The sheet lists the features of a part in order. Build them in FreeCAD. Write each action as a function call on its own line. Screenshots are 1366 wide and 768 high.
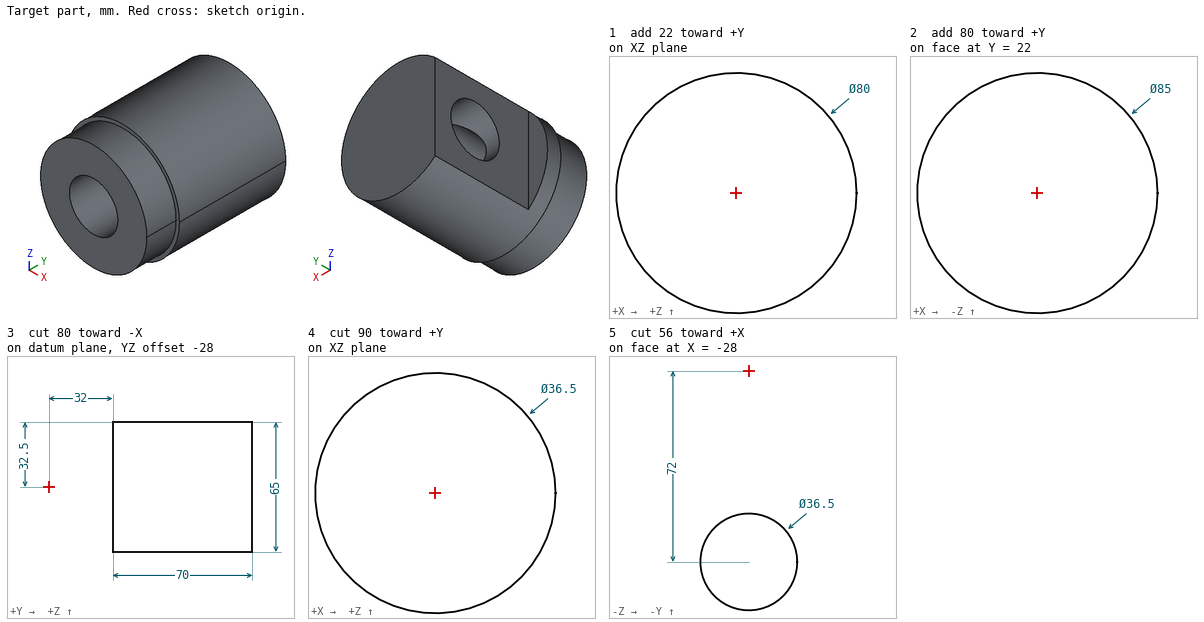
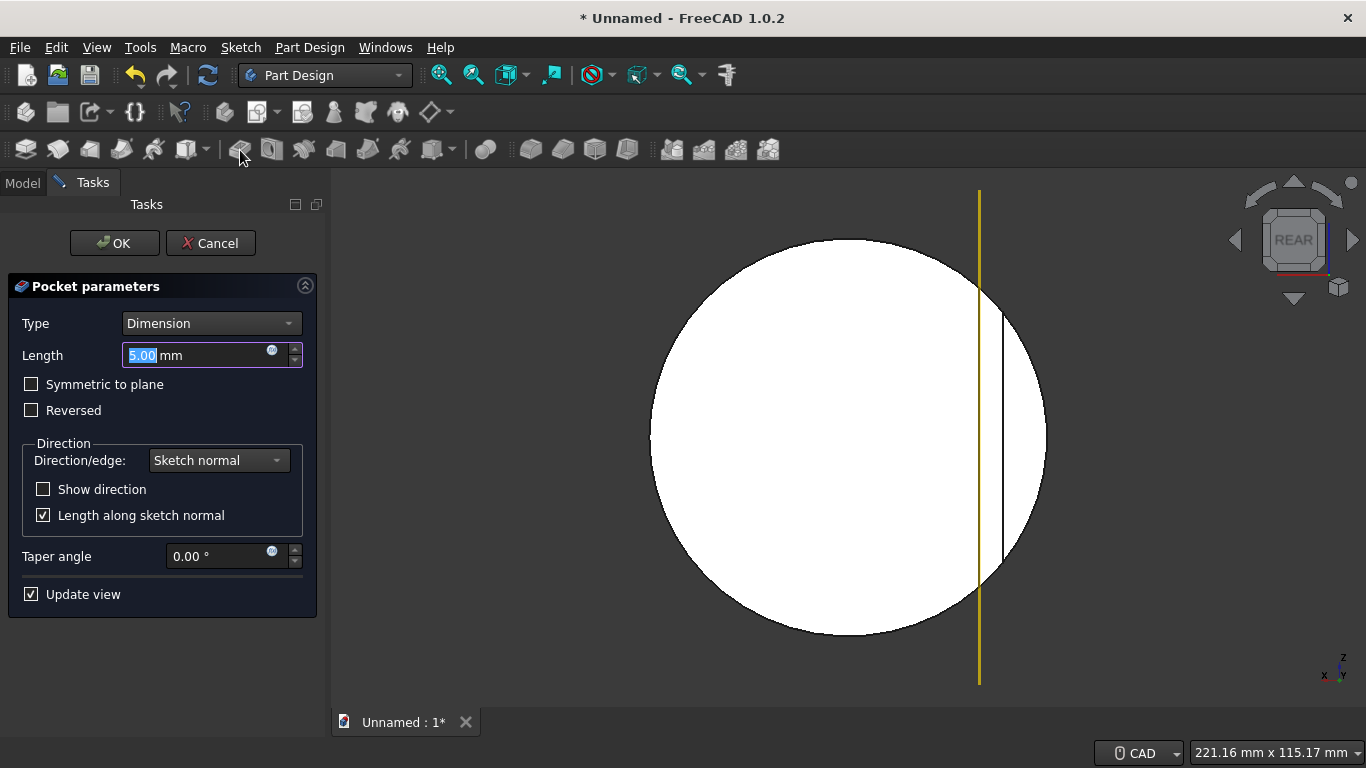
text(80)
key(Tab)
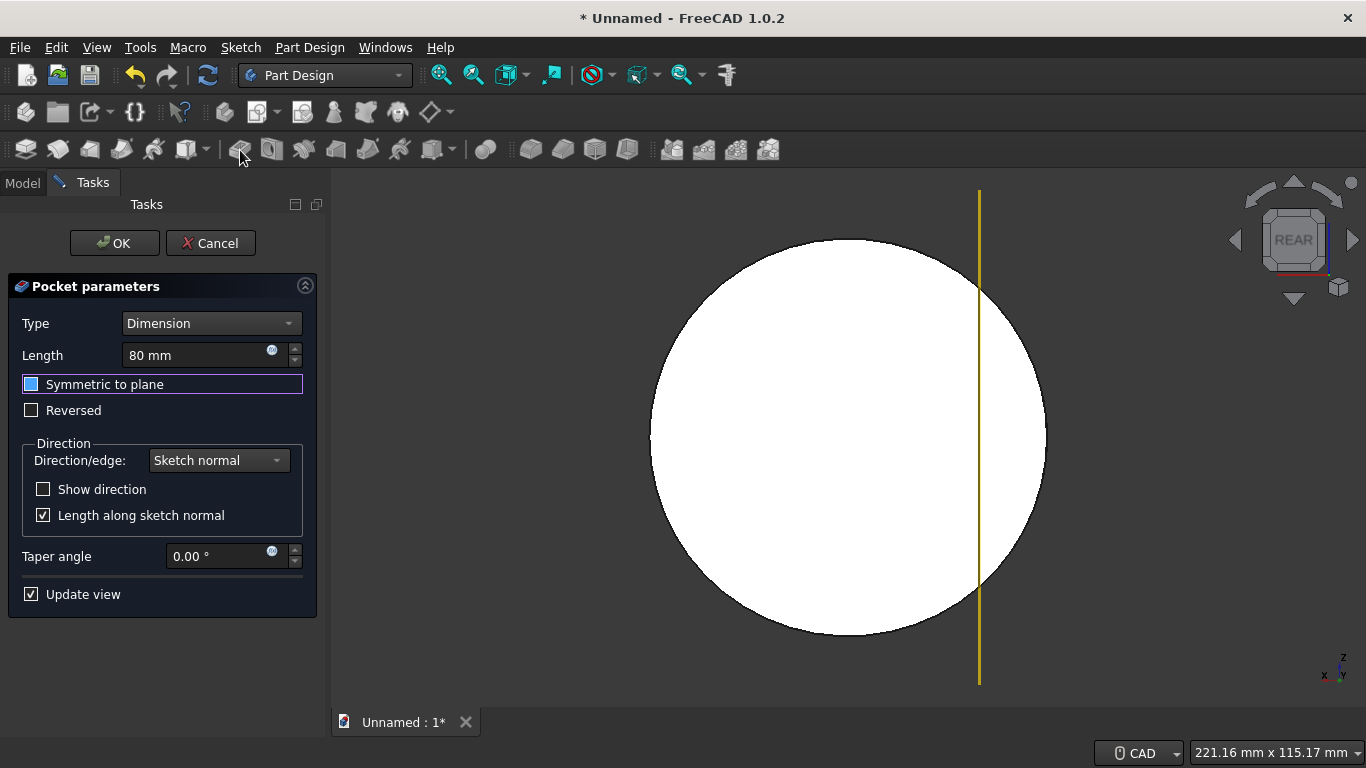
click(115, 243)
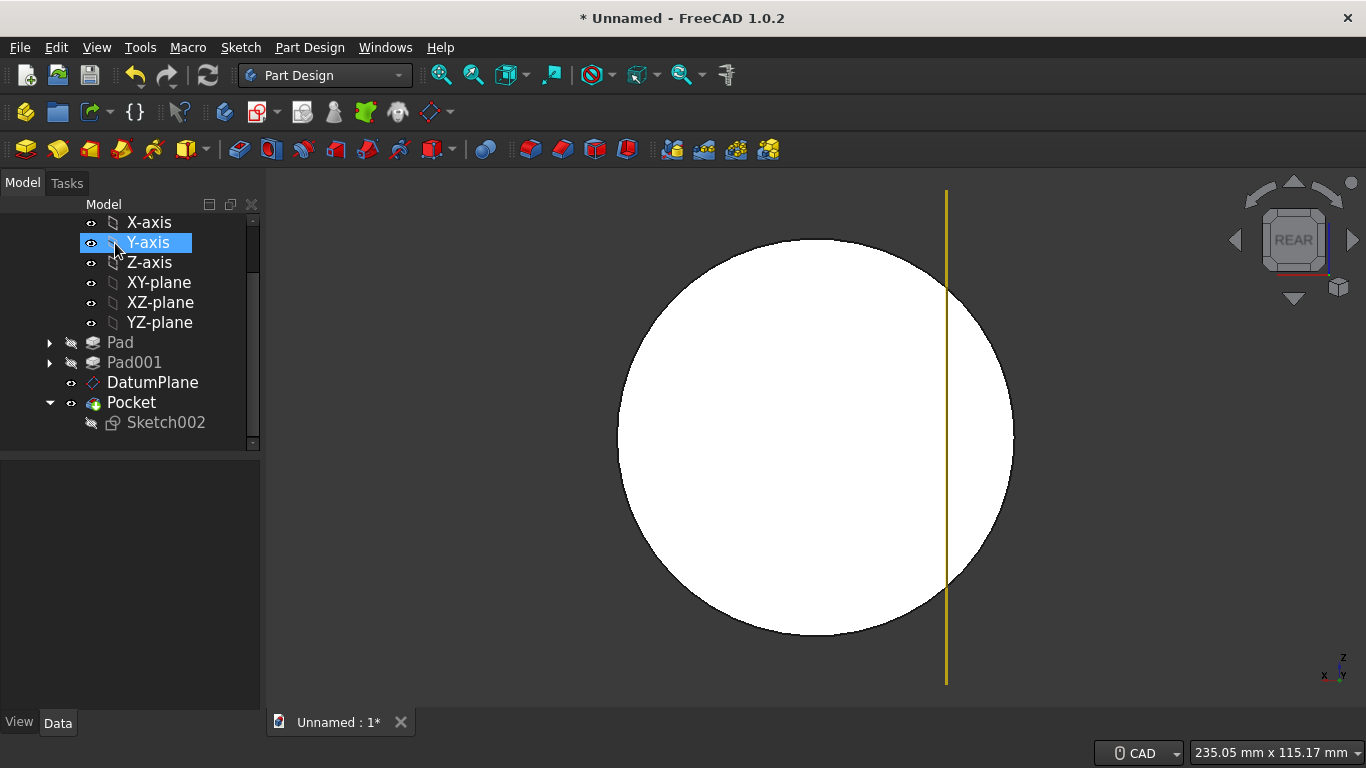
click(116, 383)
key(space)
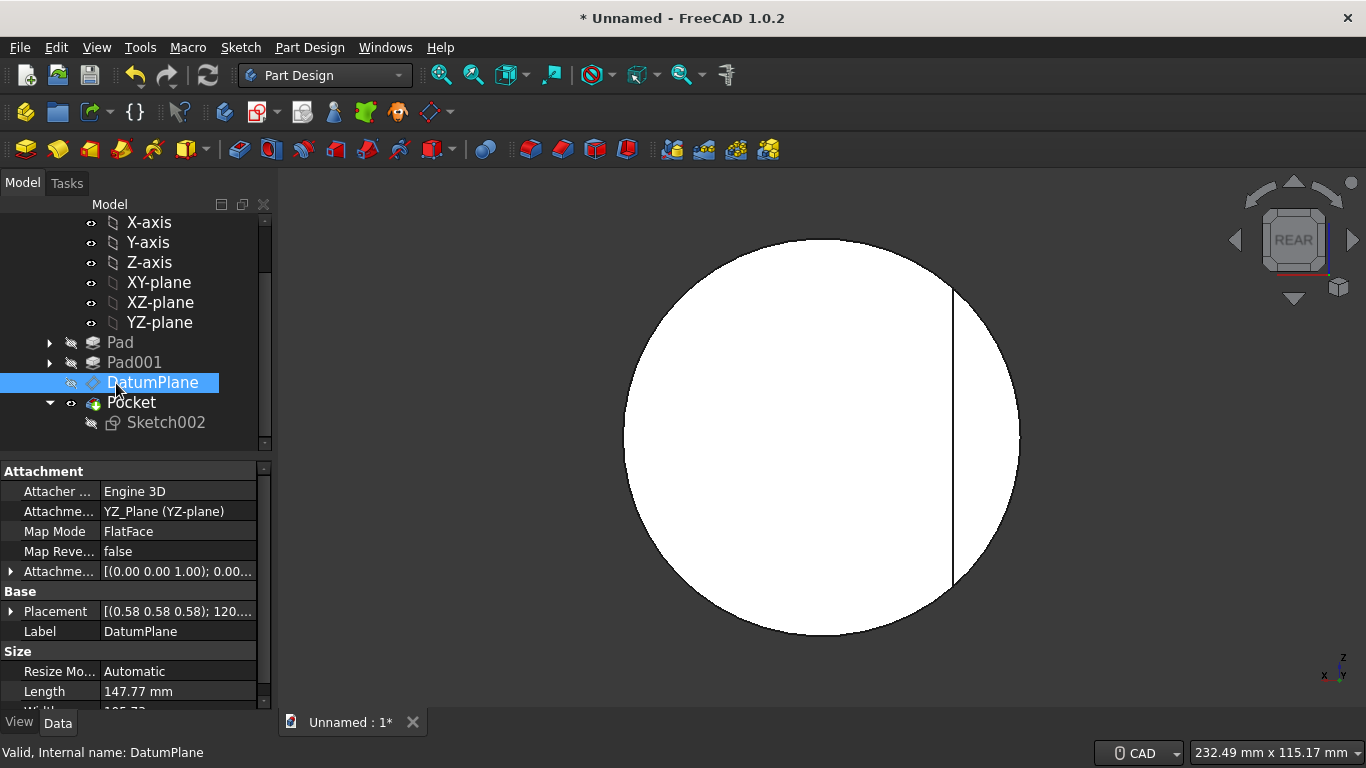
click(318, 667)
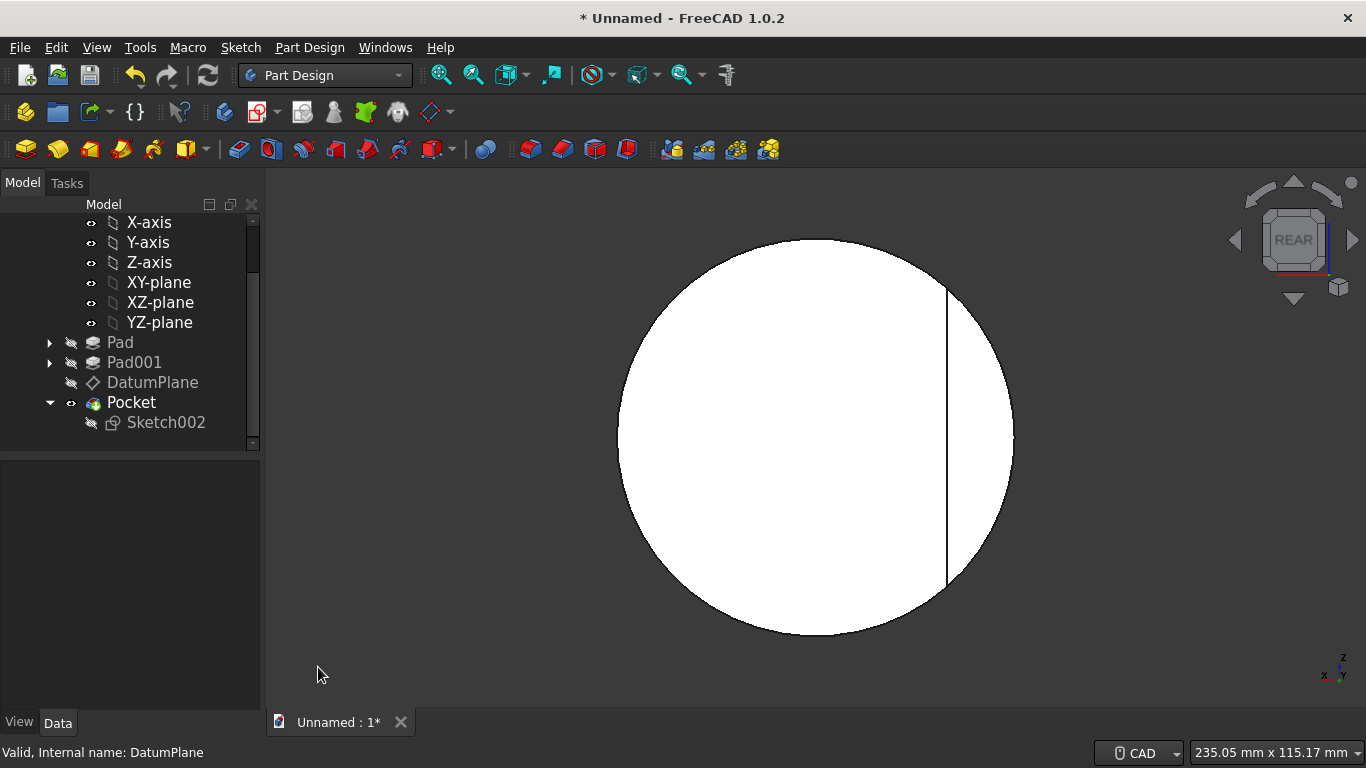
click(258, 112)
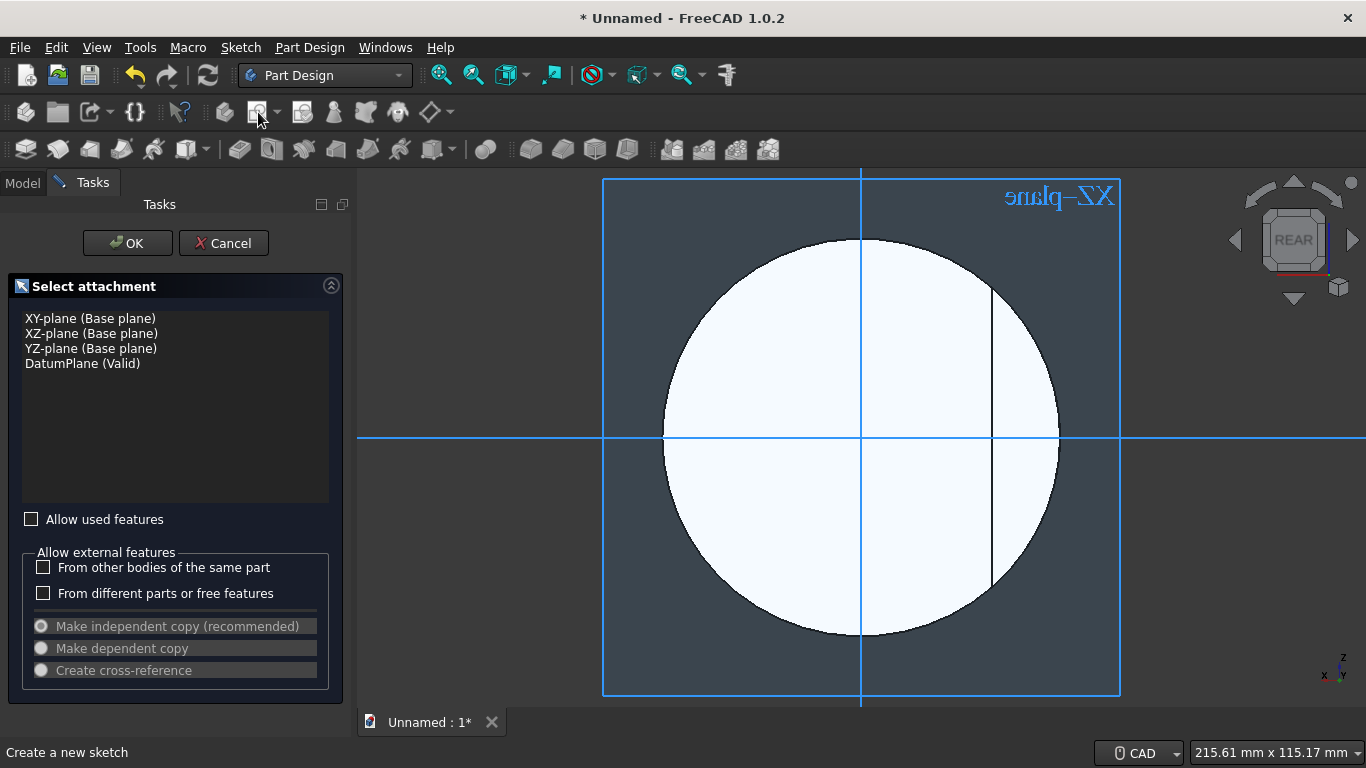
click(82, 334)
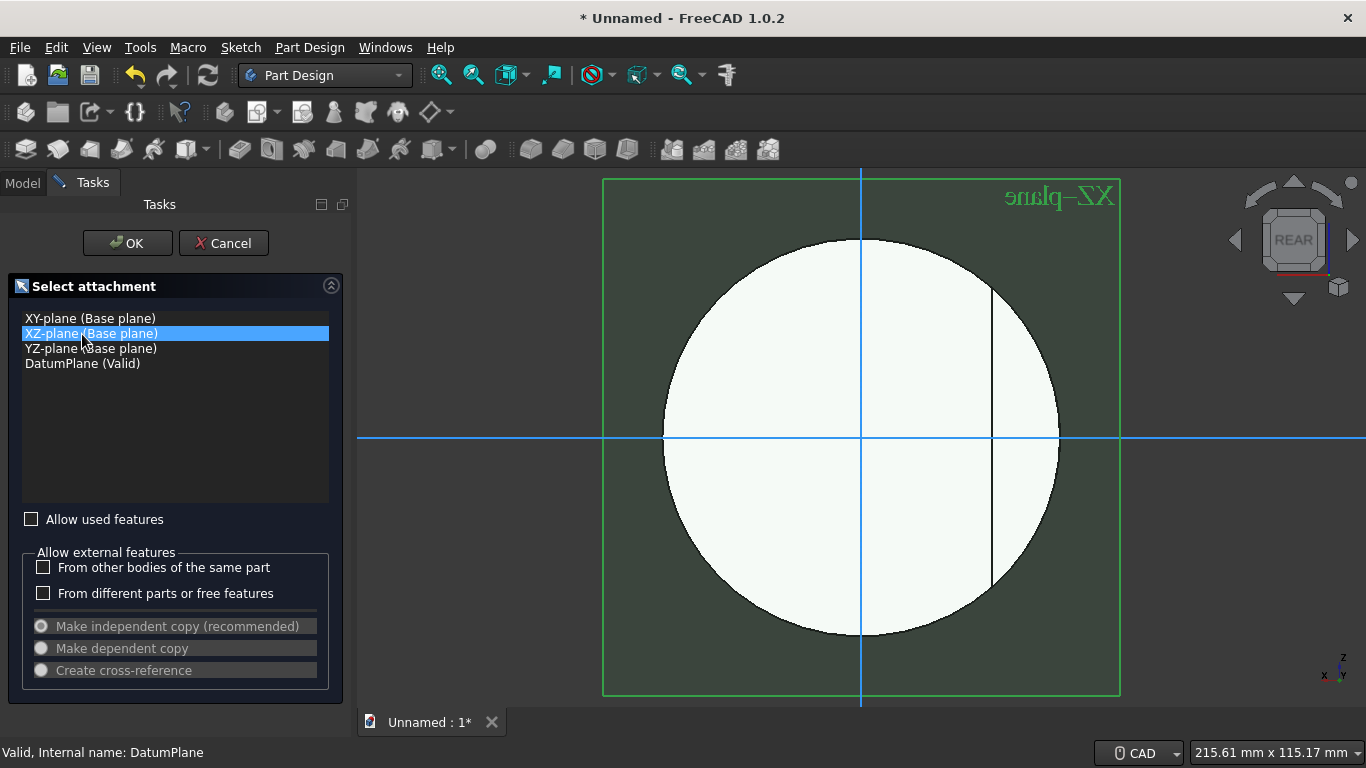
click(128, 243)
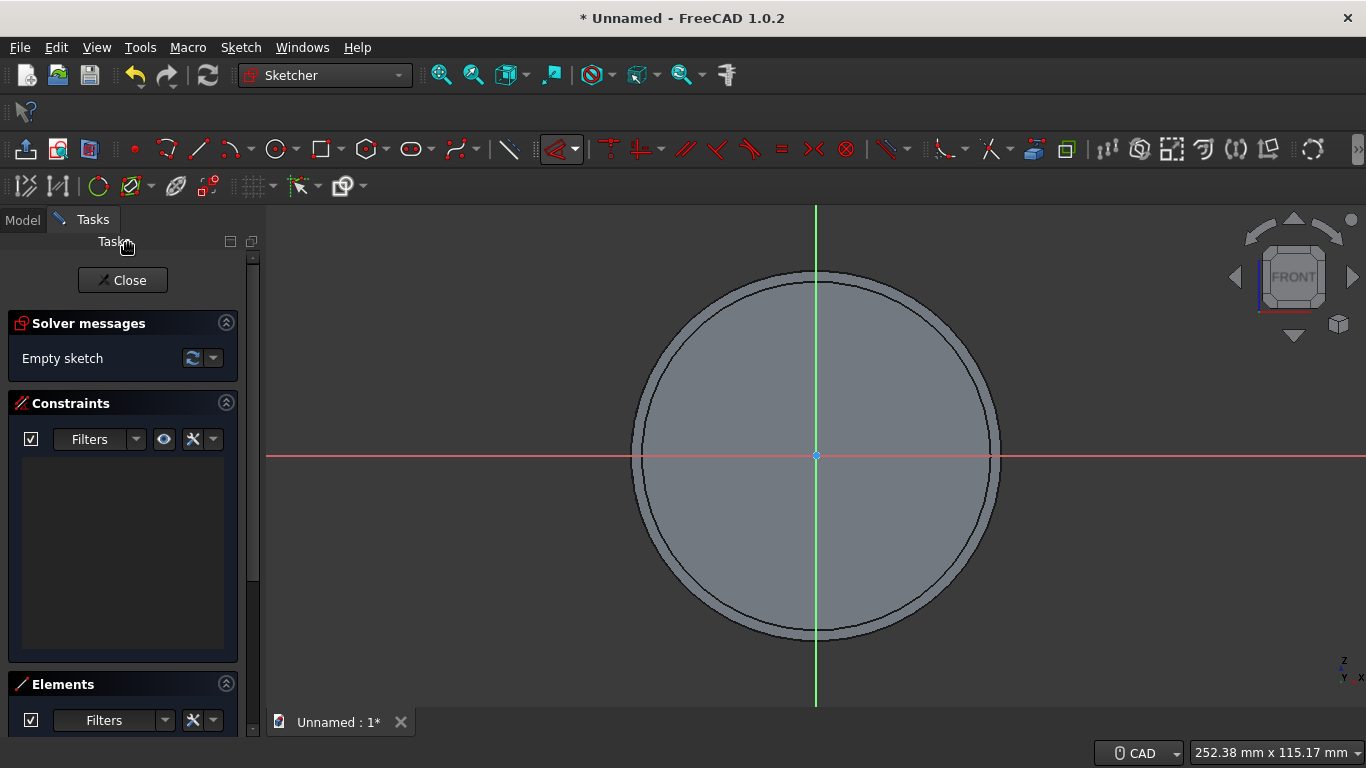
scroll(900, 456, up, 3)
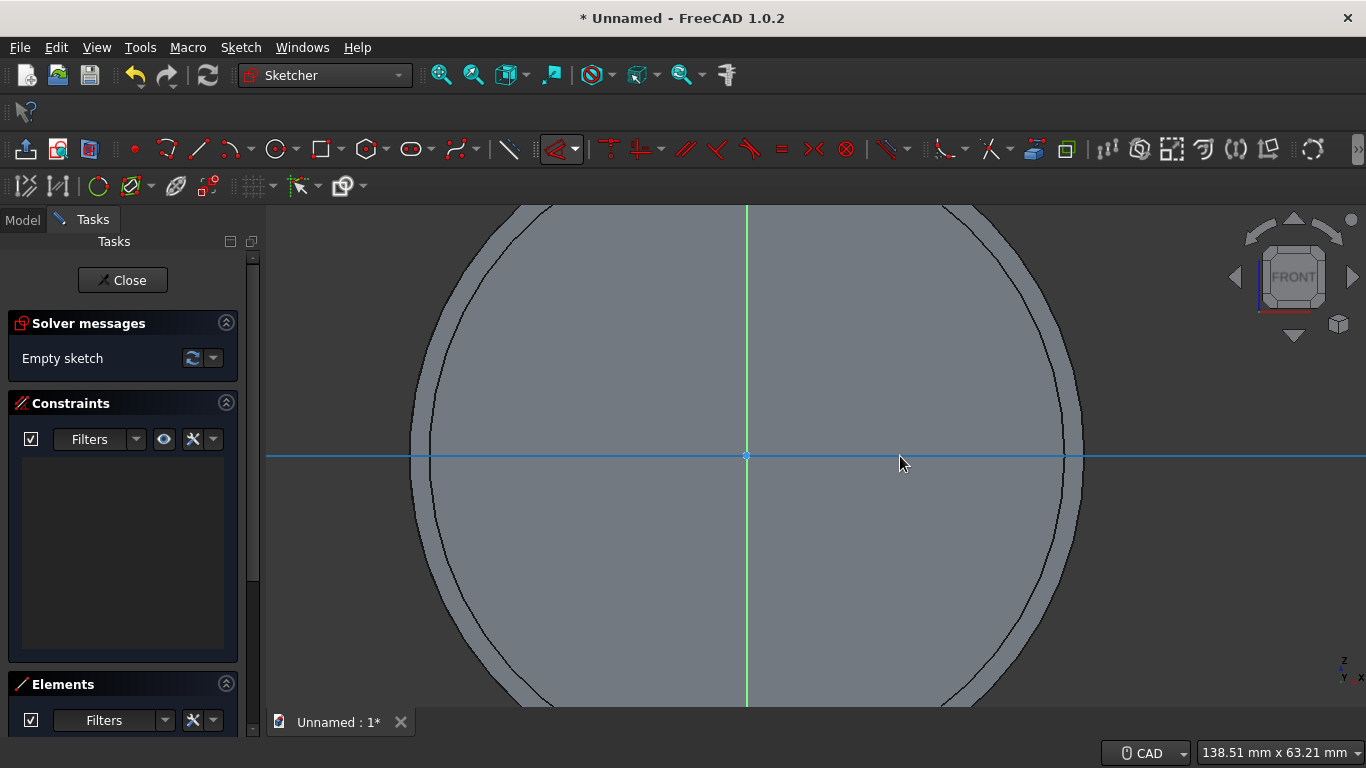
click(276, 150)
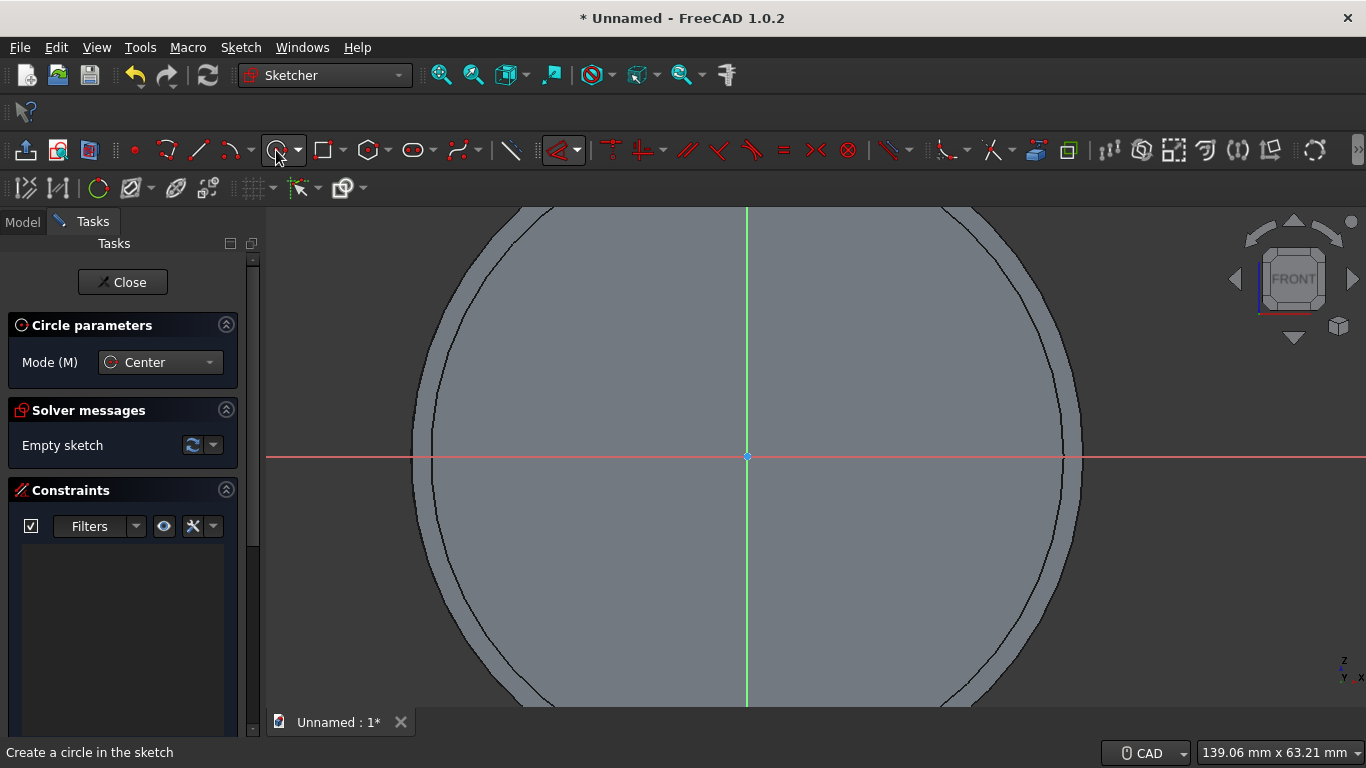
click(747, 457)
move(849, 355)